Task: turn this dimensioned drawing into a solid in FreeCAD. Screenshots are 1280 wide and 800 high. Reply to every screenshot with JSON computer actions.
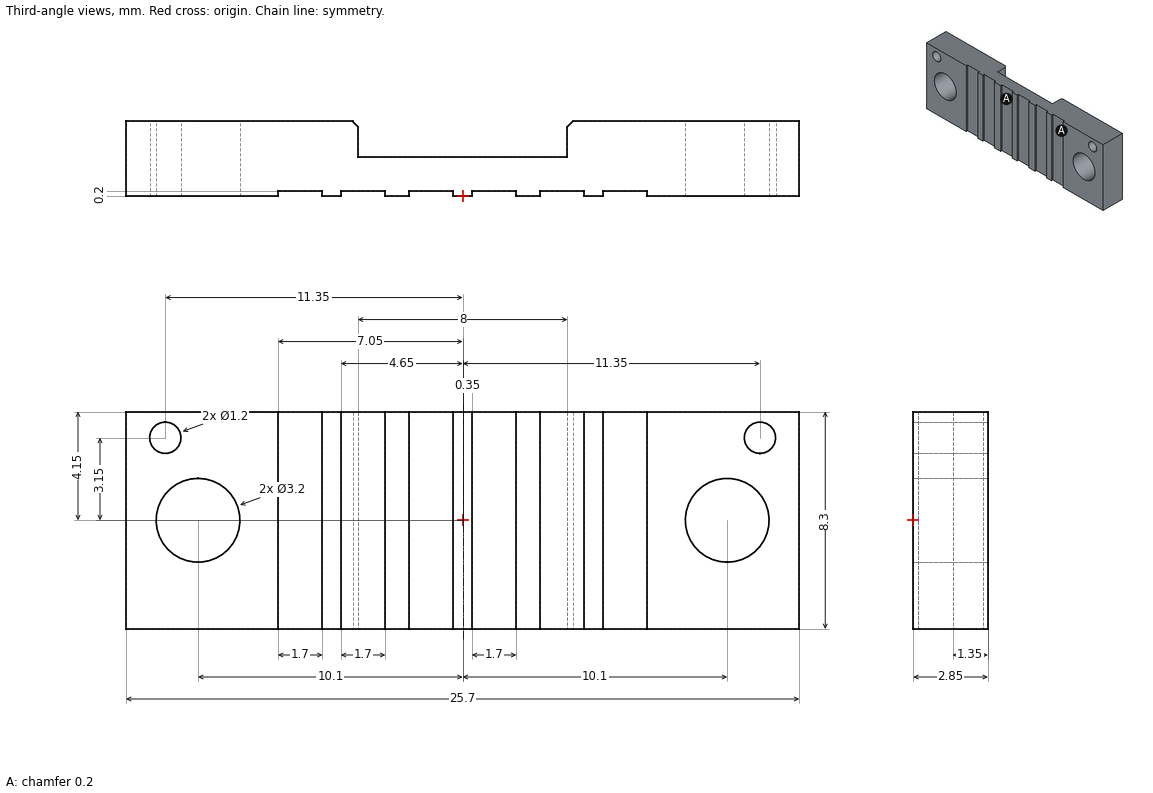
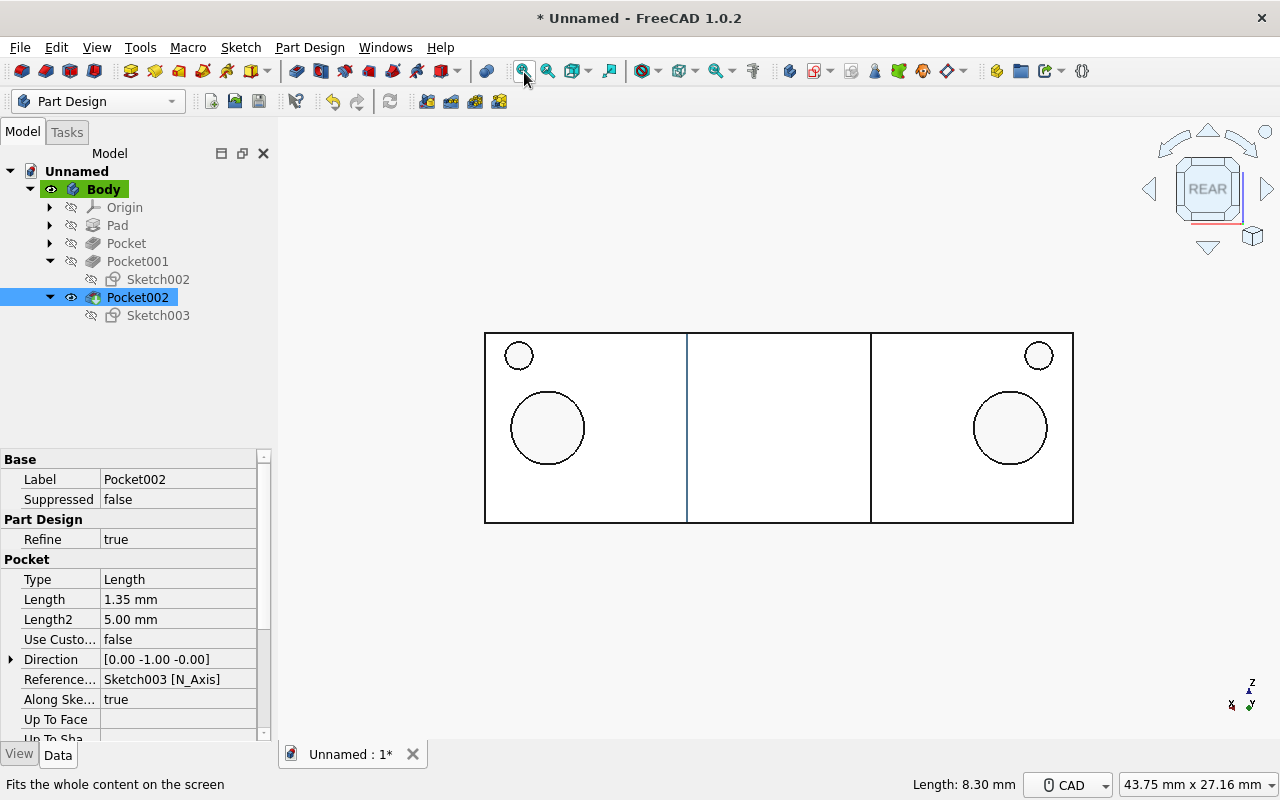
{"action": "left_click", "coordinate": [871, 427], "text": "ctrl"}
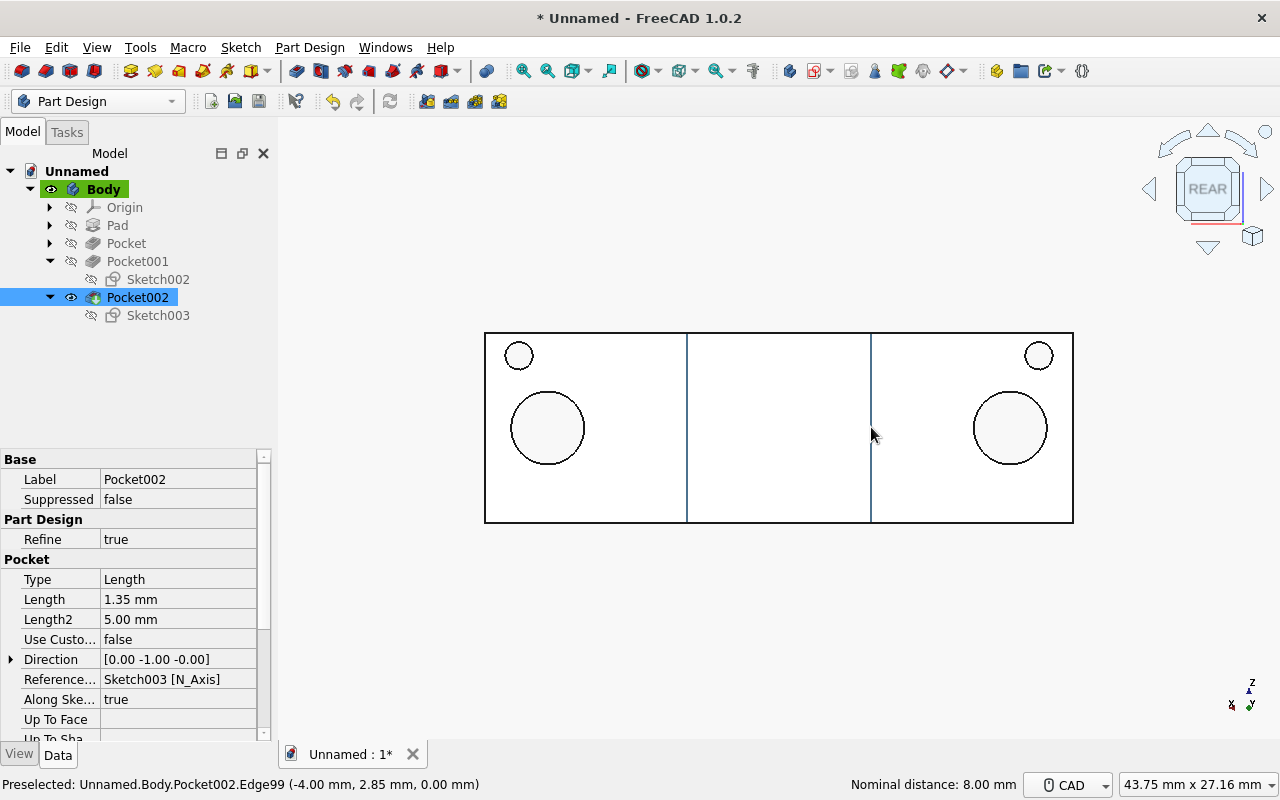
{"action": "left_click", "coordinate": [46, 72]}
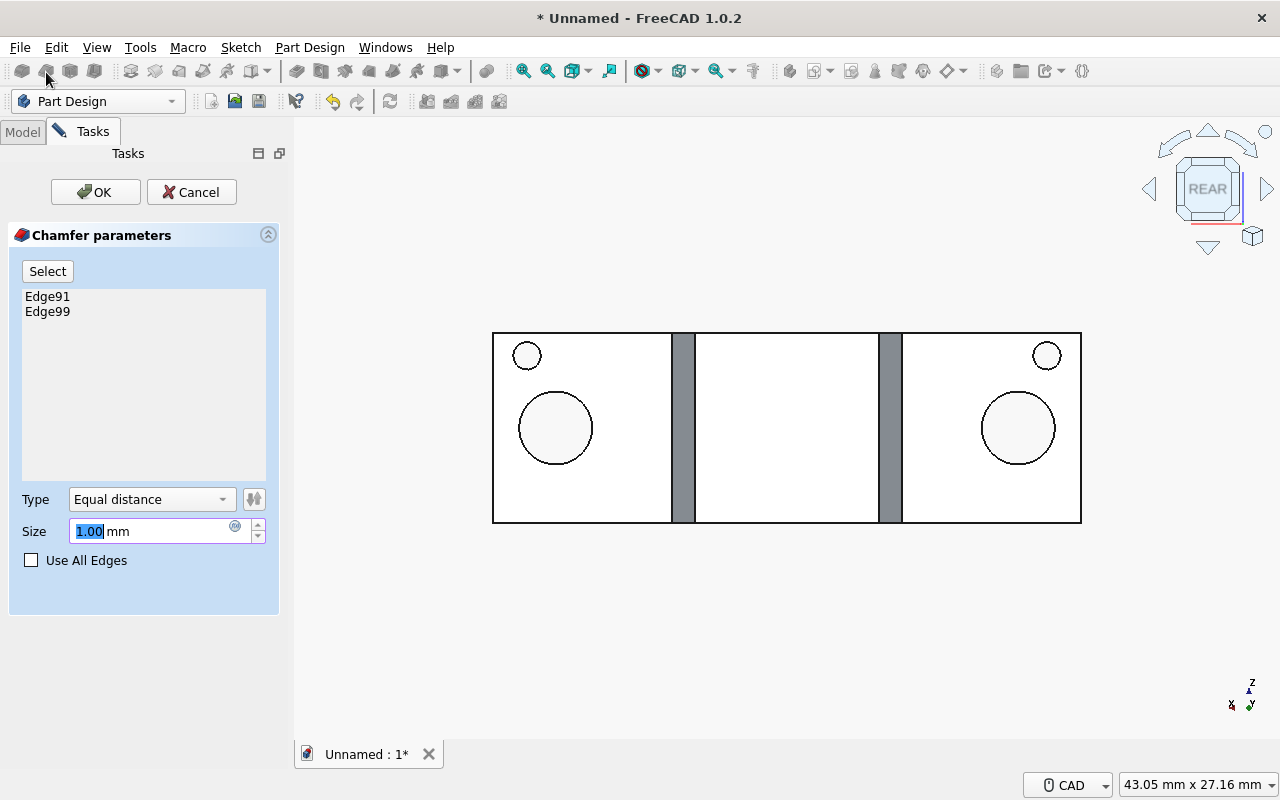
{"action": "type", "text": "0.2"}
{"action": "key", "text": "Tab"}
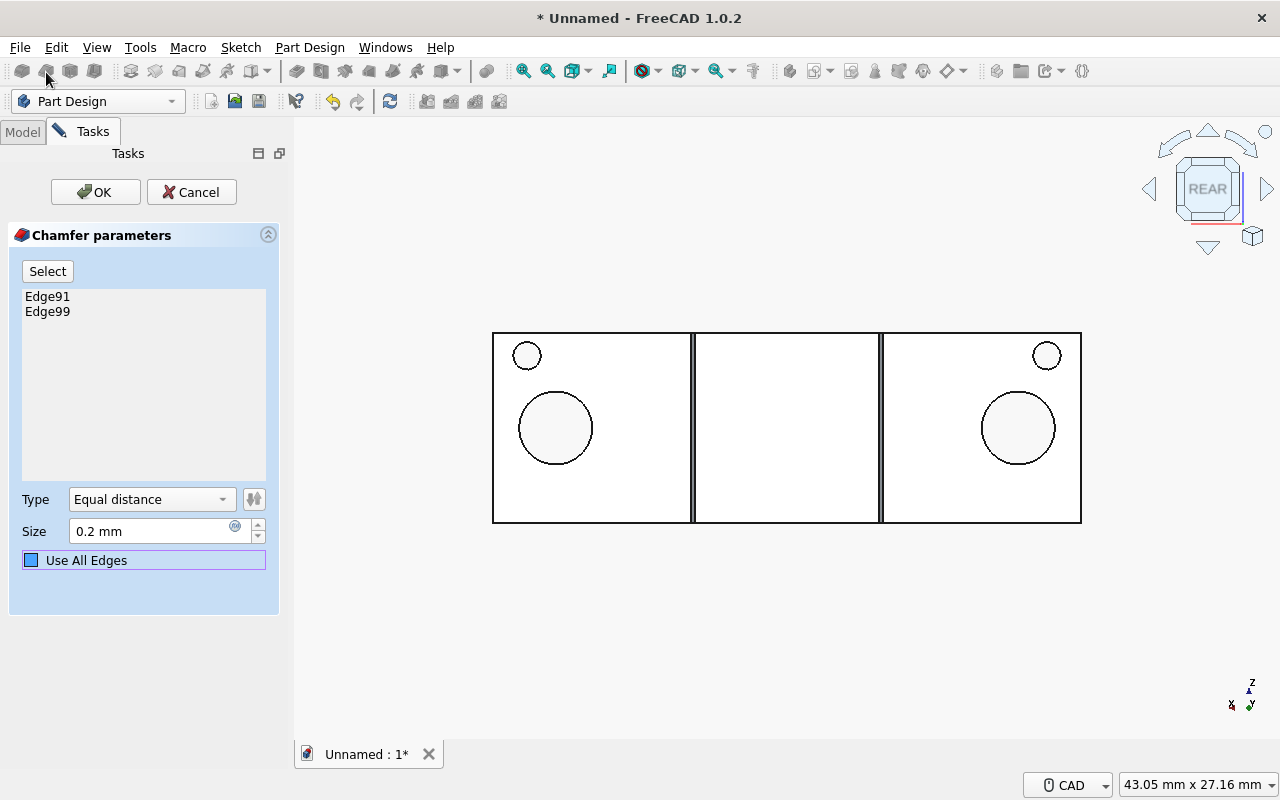
{"action": "left_click", "coordinate": [96, 192]}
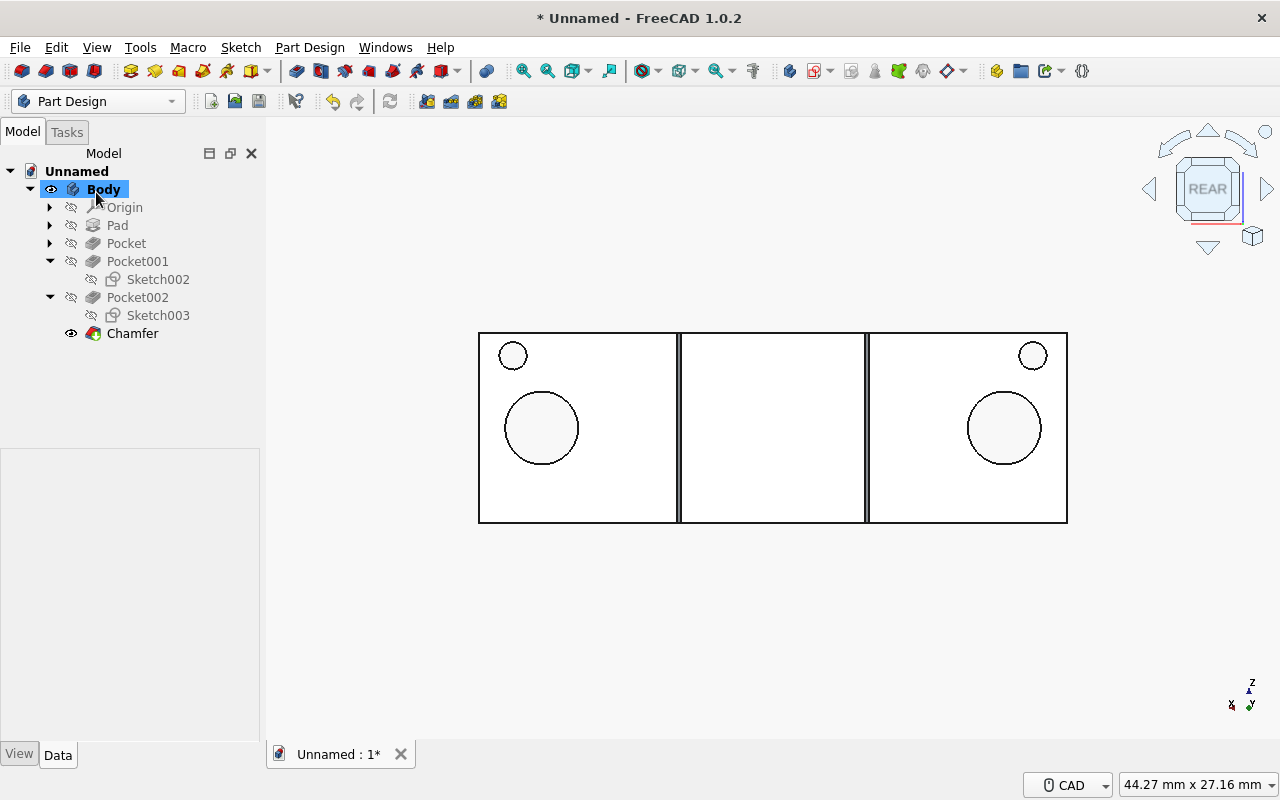
{"action": "key", "text": "0"}